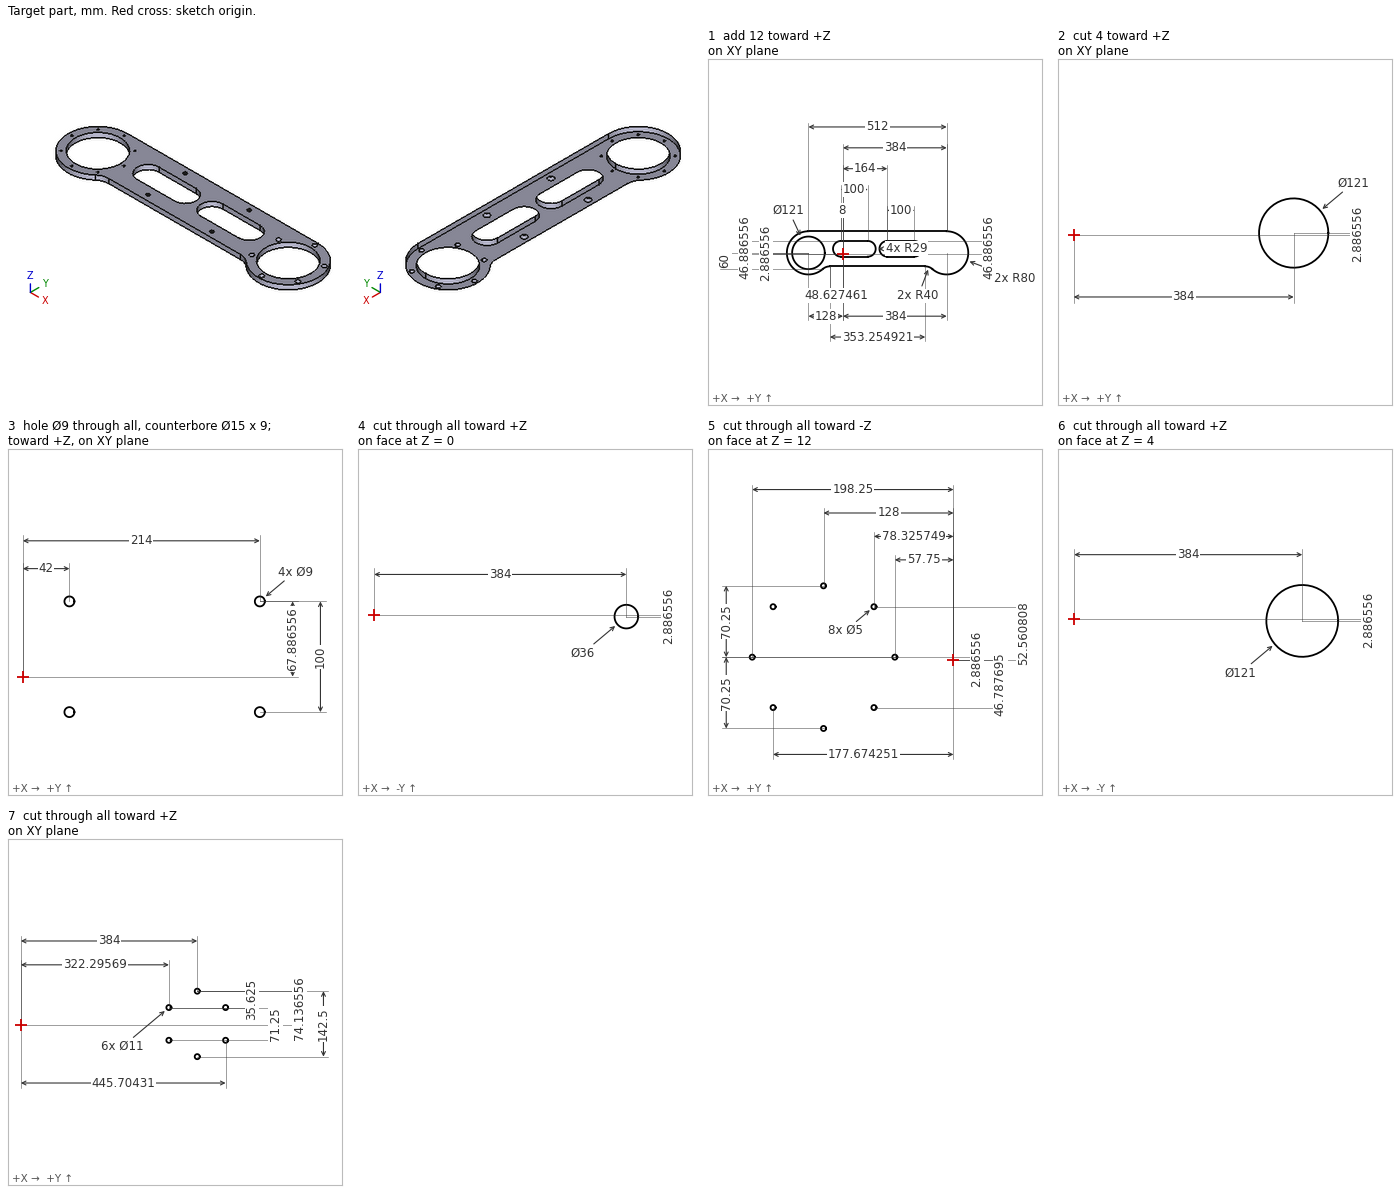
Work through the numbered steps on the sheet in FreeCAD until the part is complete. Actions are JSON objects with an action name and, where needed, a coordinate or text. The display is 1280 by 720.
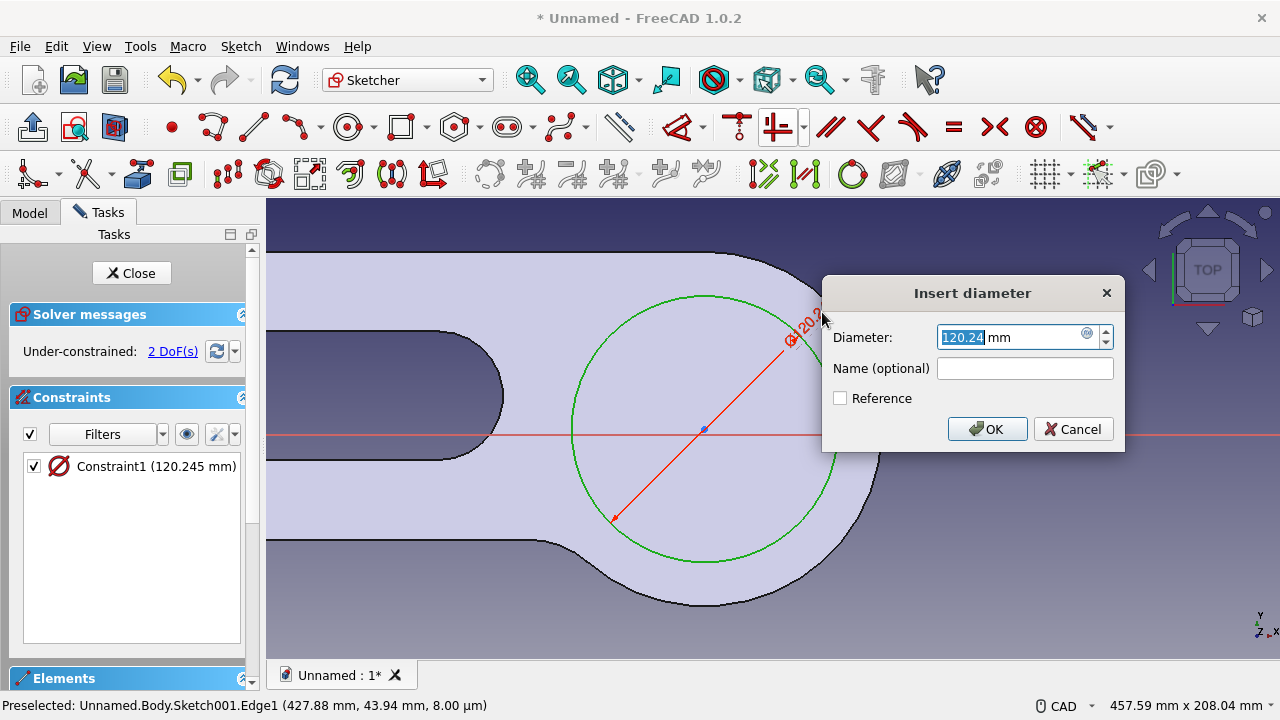
{"action": "type", "text": "121"}
{"action": "key", "text": "Return"}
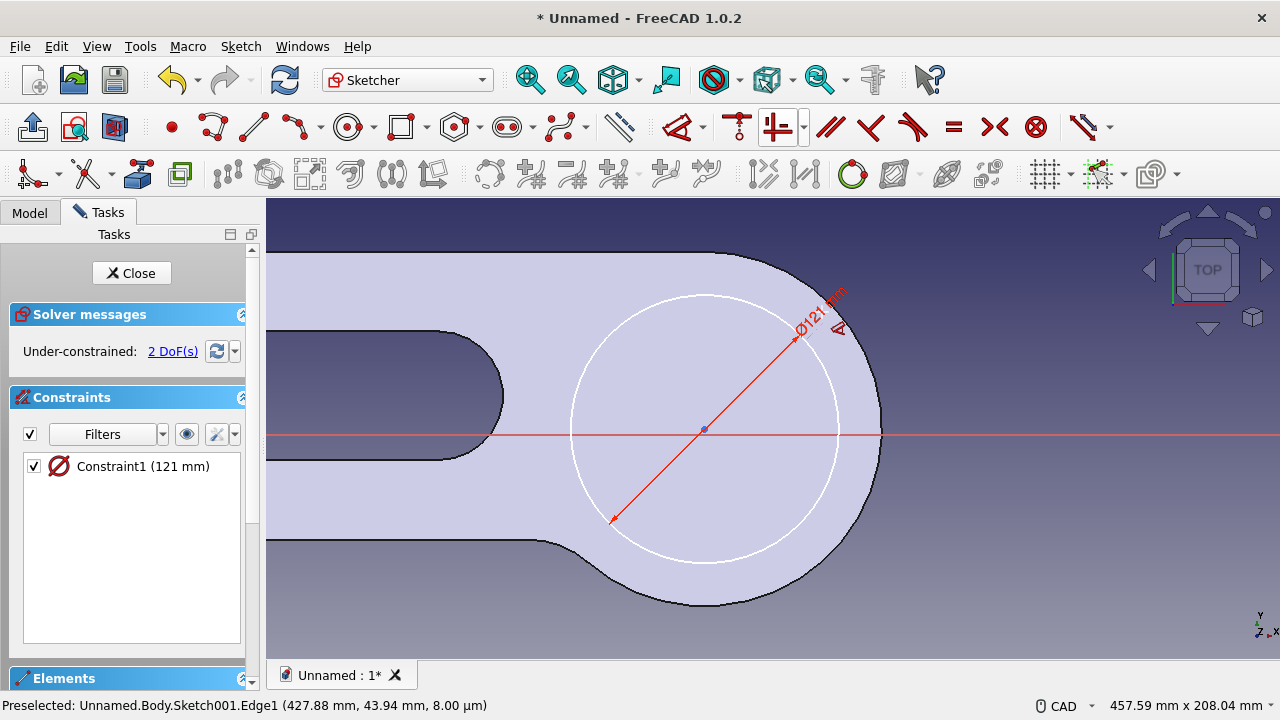
{"action": "left_click", "coordinate": [705, 429]}
{"action": "left_click", "coordinate": [499, 469]}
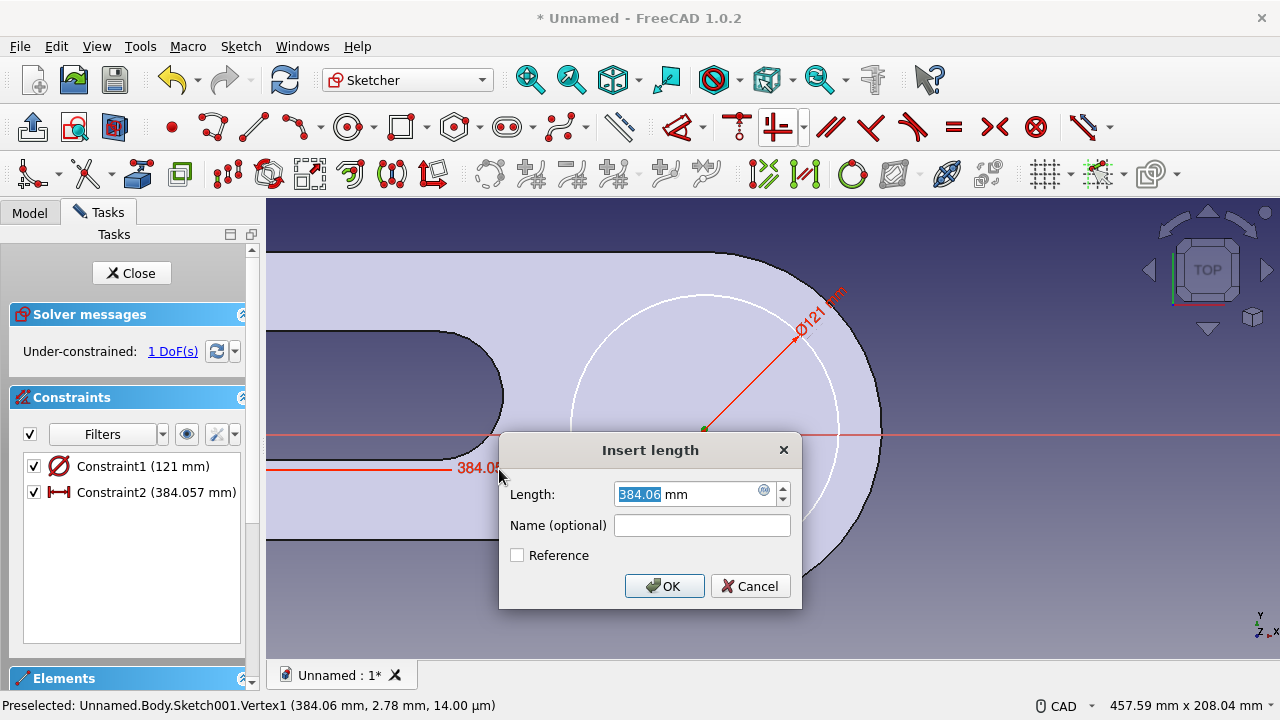
{"action": "type", "text": "384"}
{"action": "key", "text": "Return"}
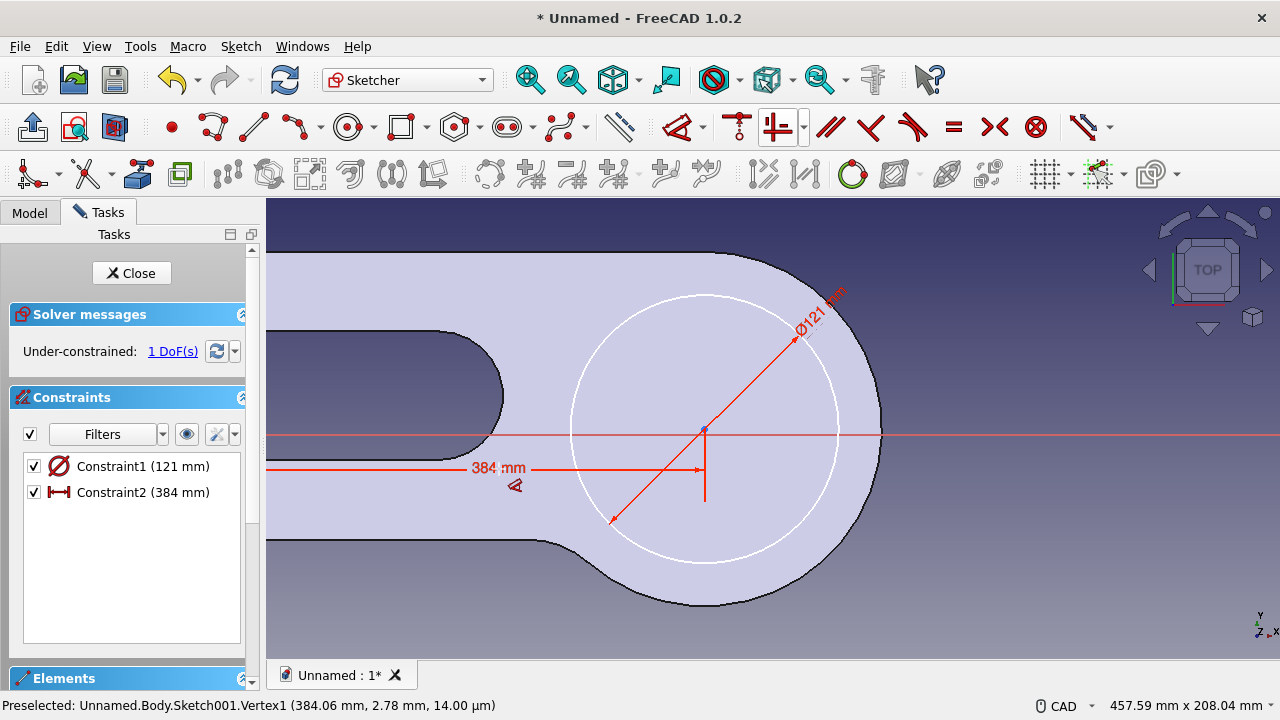
{"action": "scroll", "coordinate": [705, 429], "scroll_direction": "up", "scroll_amount": 10}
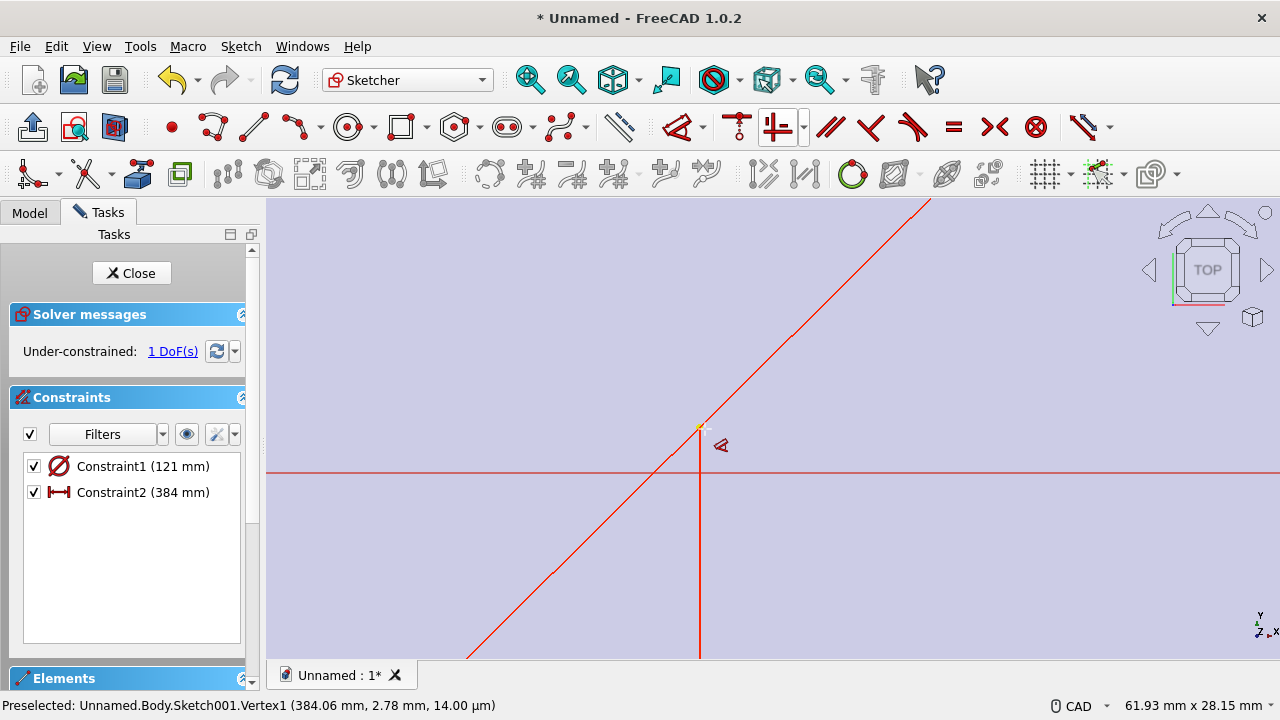
{"action": "left_click", "coordinate": [700, 427]}
{"action": "left_click", "coordinate": [734, 450]}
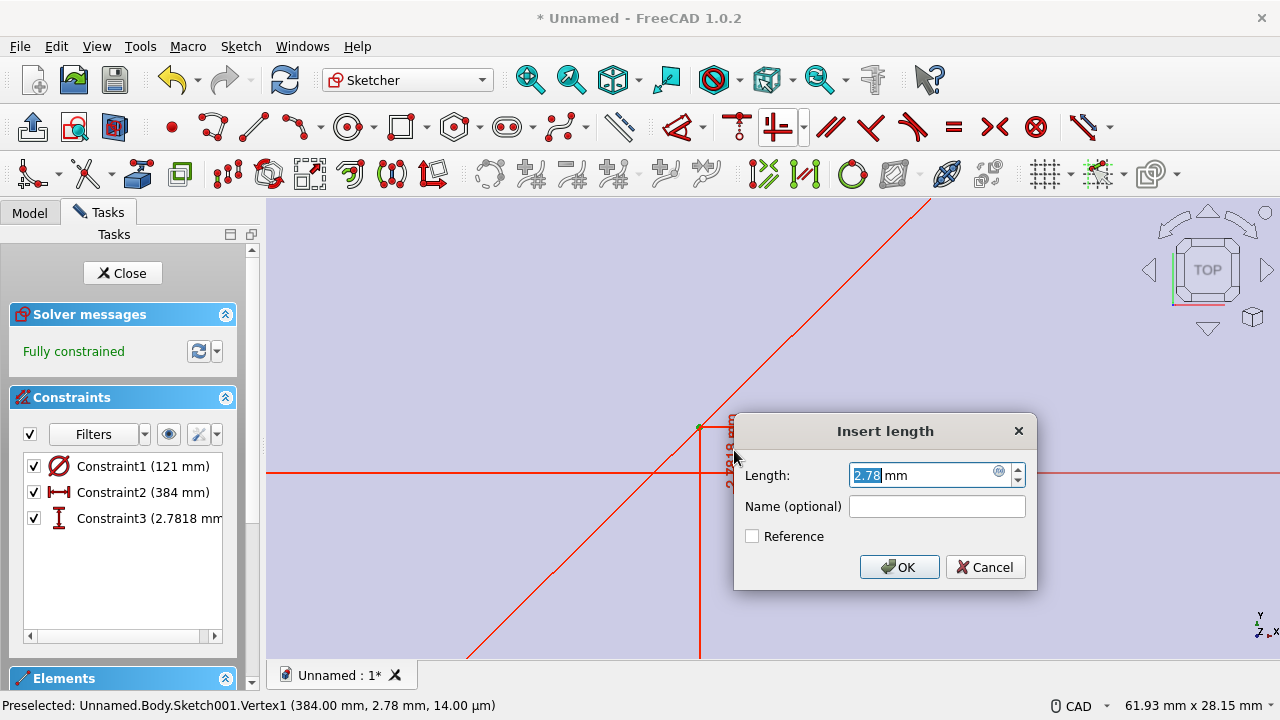
{"action": "type", "text": "2.886556"}
{"action": "key", "text": "Return"}
{"action": "key", "text": "Escape"}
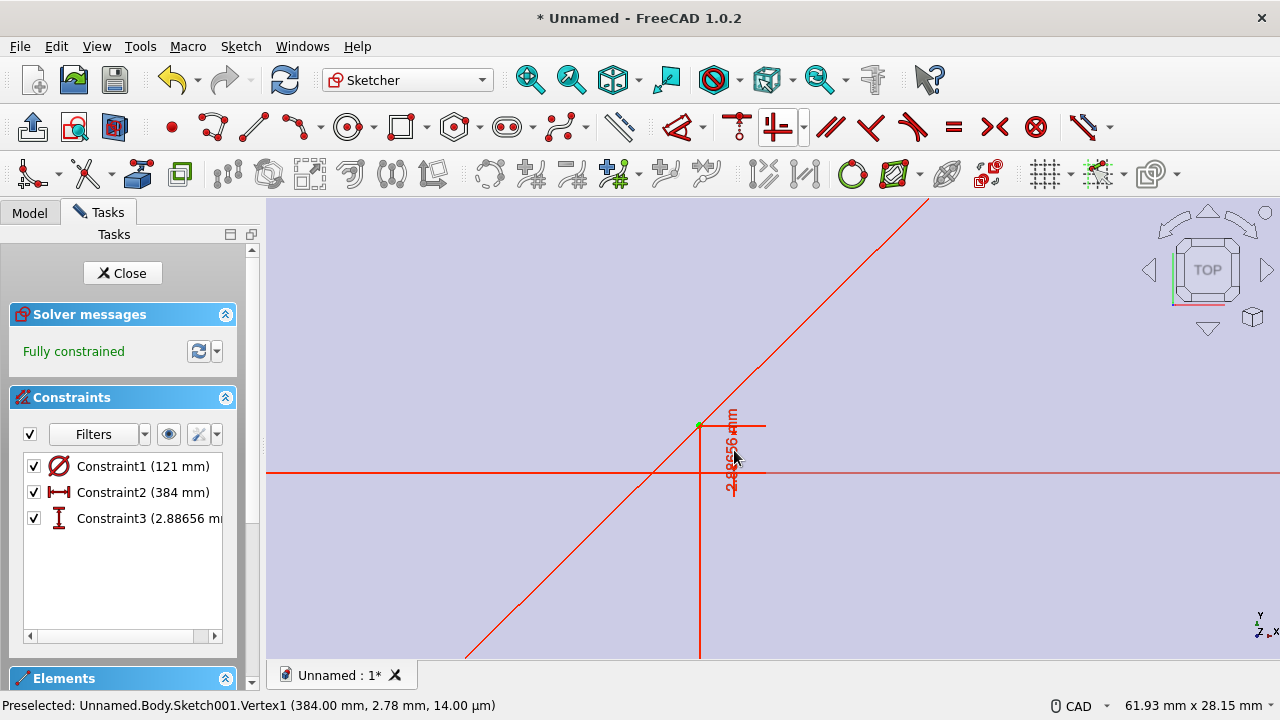
{"action": "left_click", "coordinate": [123, 273]}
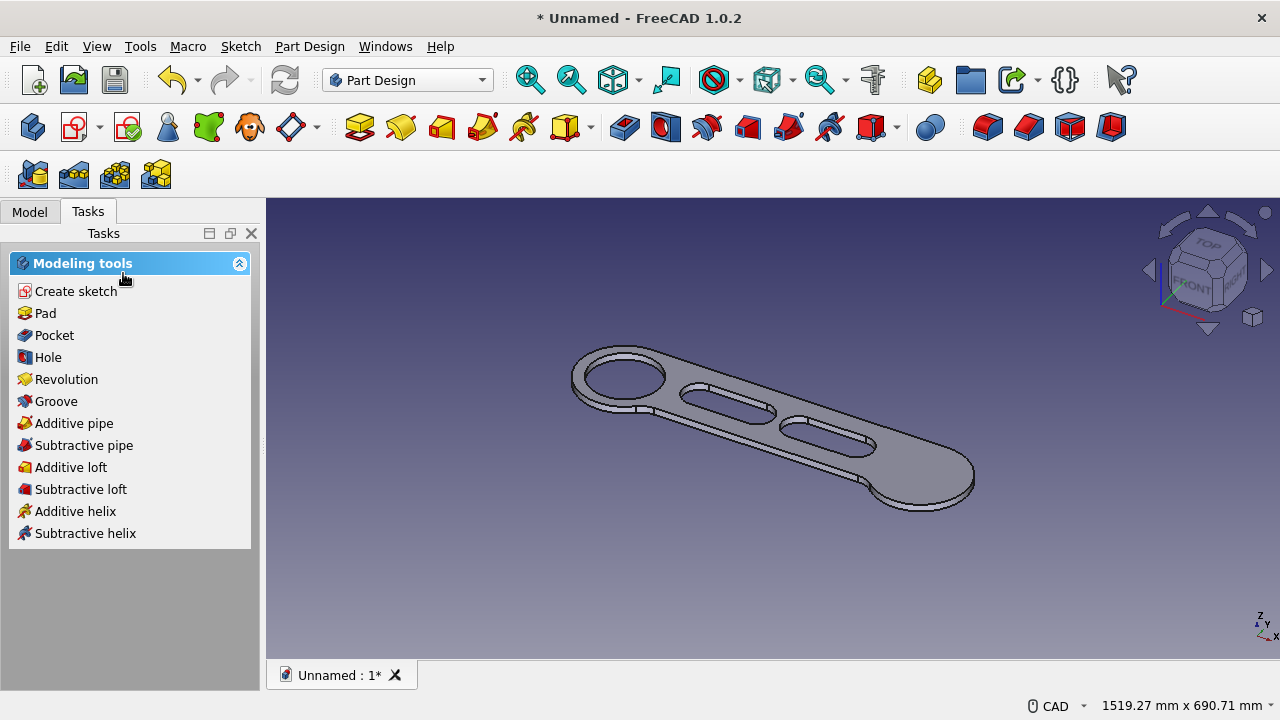
{"action": "left_click", "coordinate": [625, 128]}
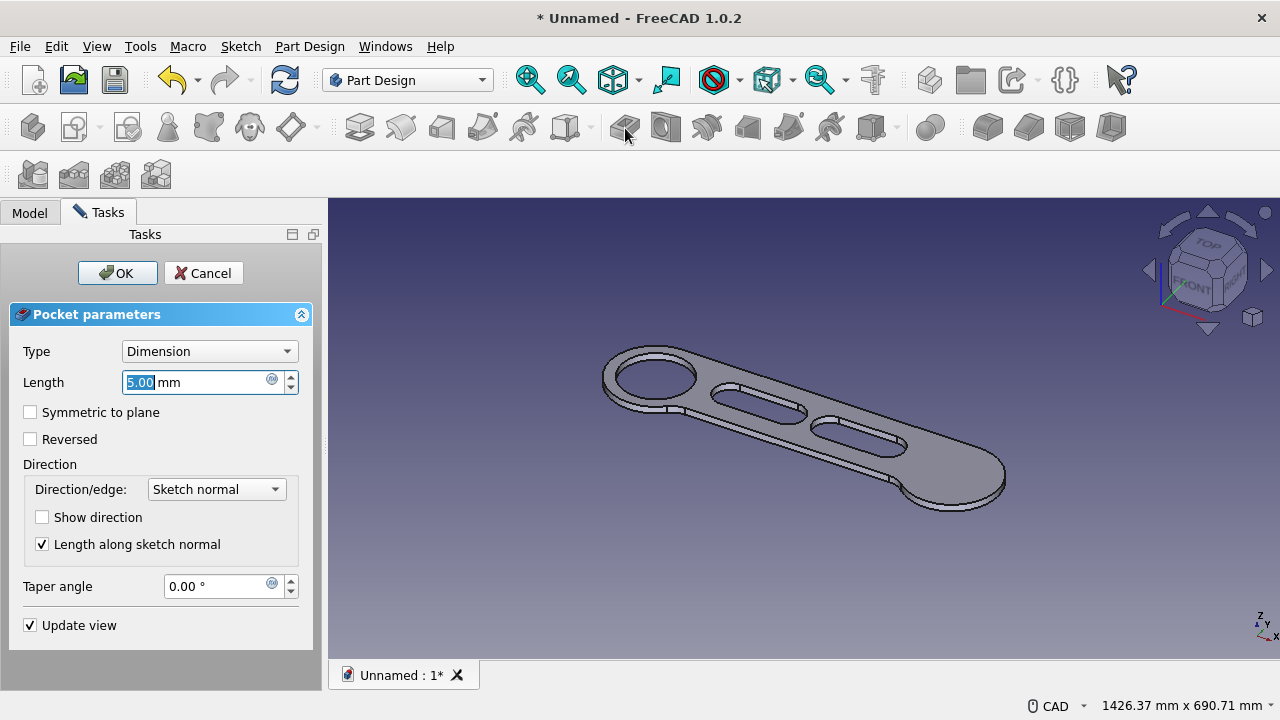
{"action": "type", "text": "4"}
{"action": "key", "text": "Tab"}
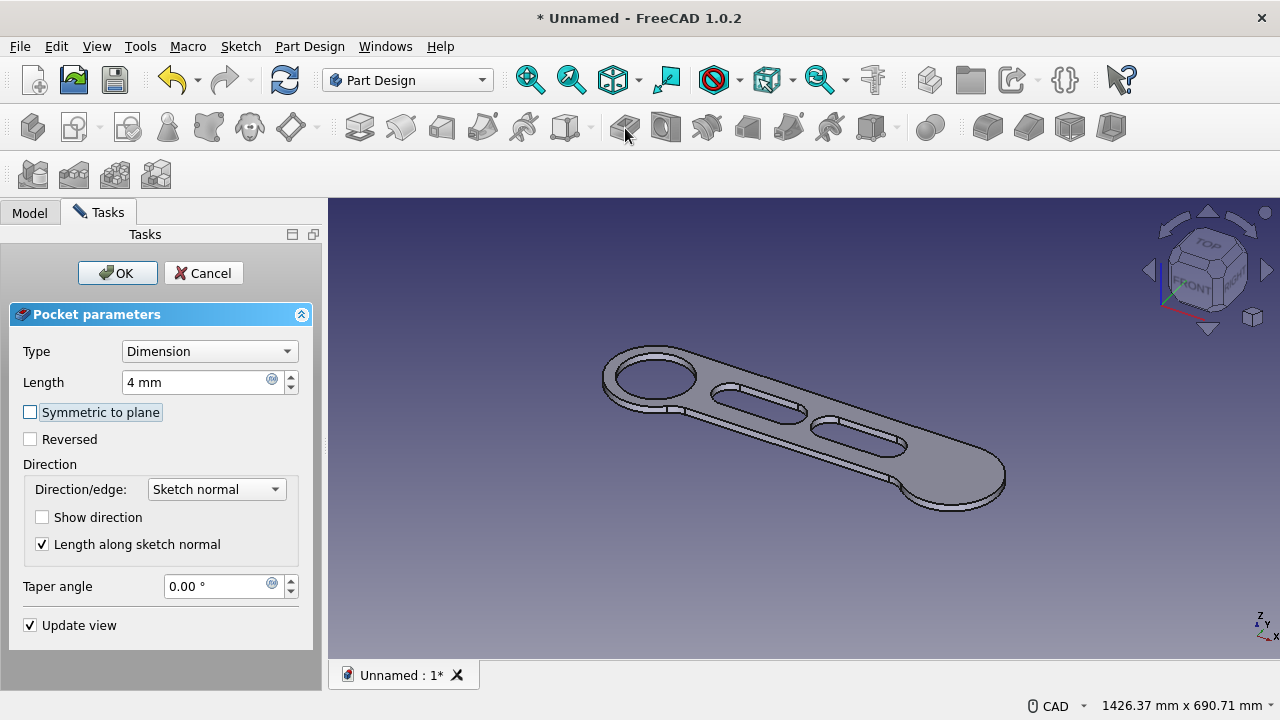
{"action": "left_click", "coordinate": [31, 439]}